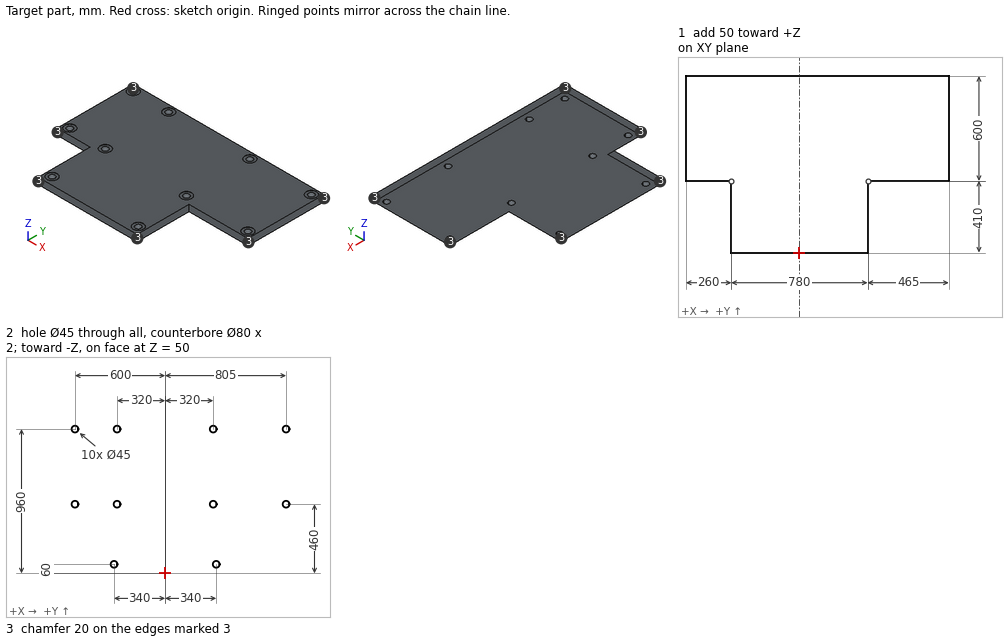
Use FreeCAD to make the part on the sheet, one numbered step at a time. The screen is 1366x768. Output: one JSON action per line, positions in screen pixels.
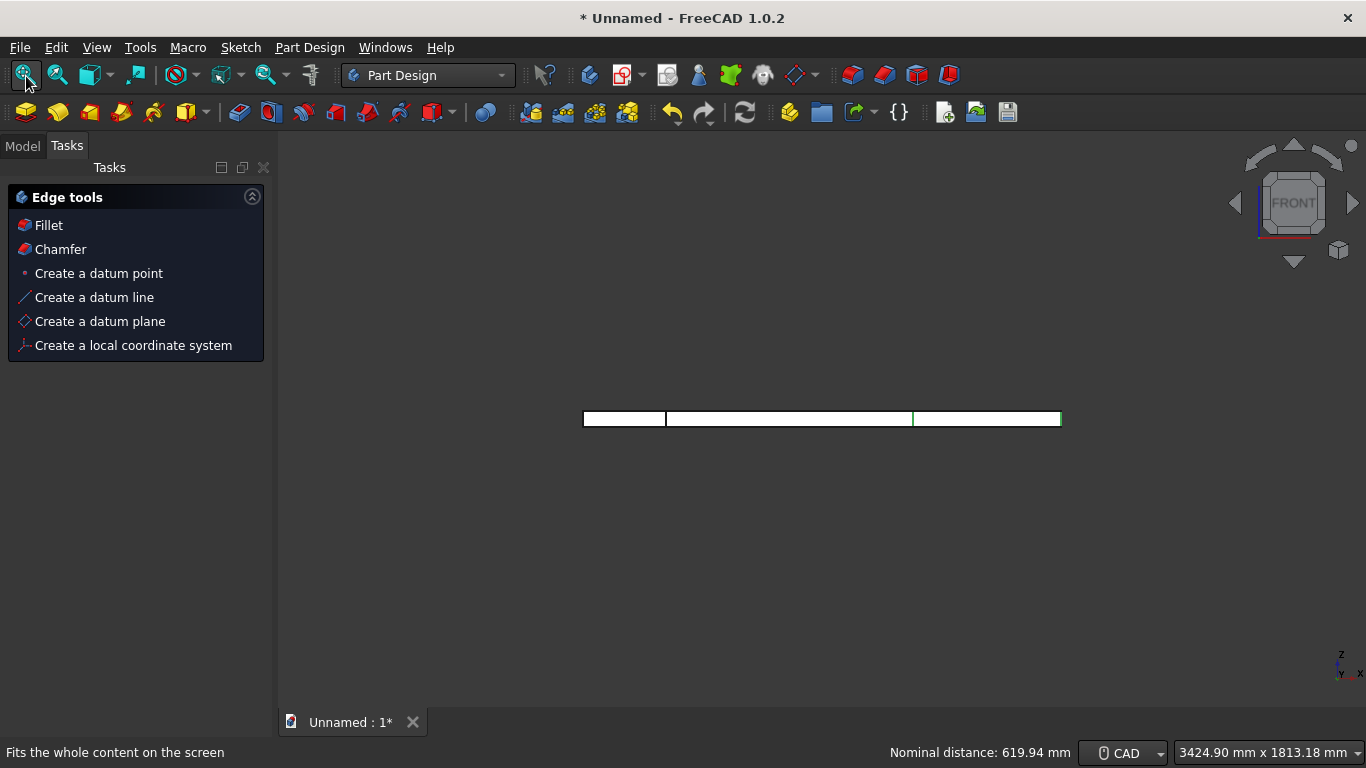
{"action": "key", "text": "v f"}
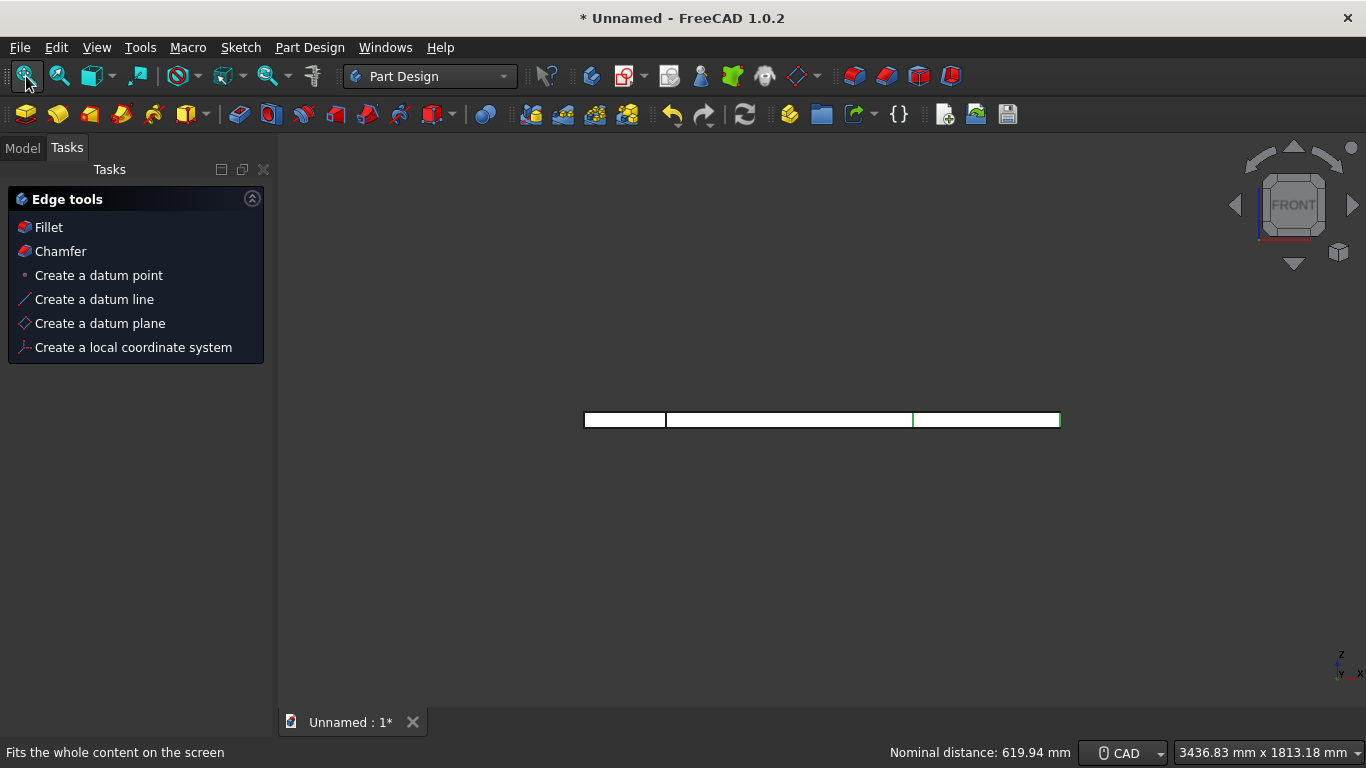
{"action": "left_click", "coordinate": [584, 419], "text": "ctrl"}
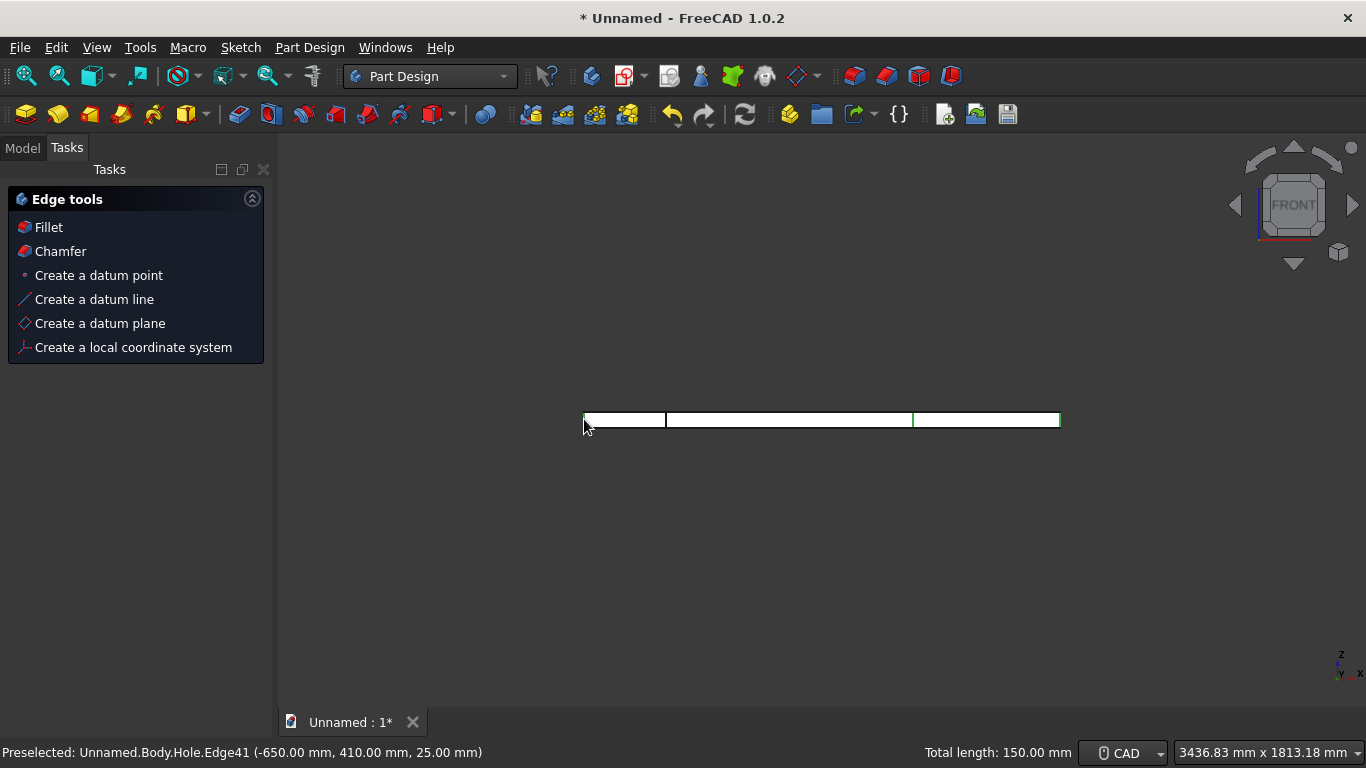
{"action": "scroll", "coordinate": [584, 419], "scroll_direction": "up", "scroll_amount": 5}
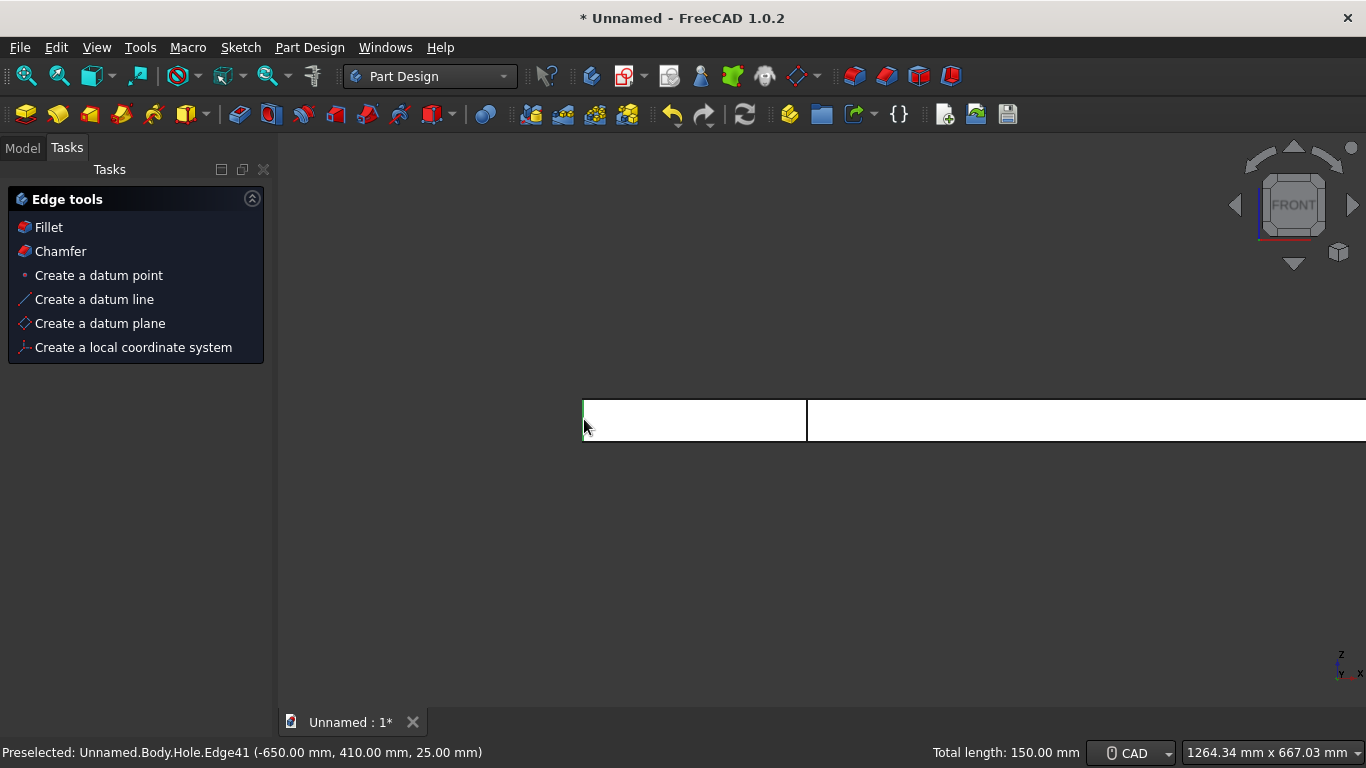
{"action": "left_click", "coordinate": [28, 76]}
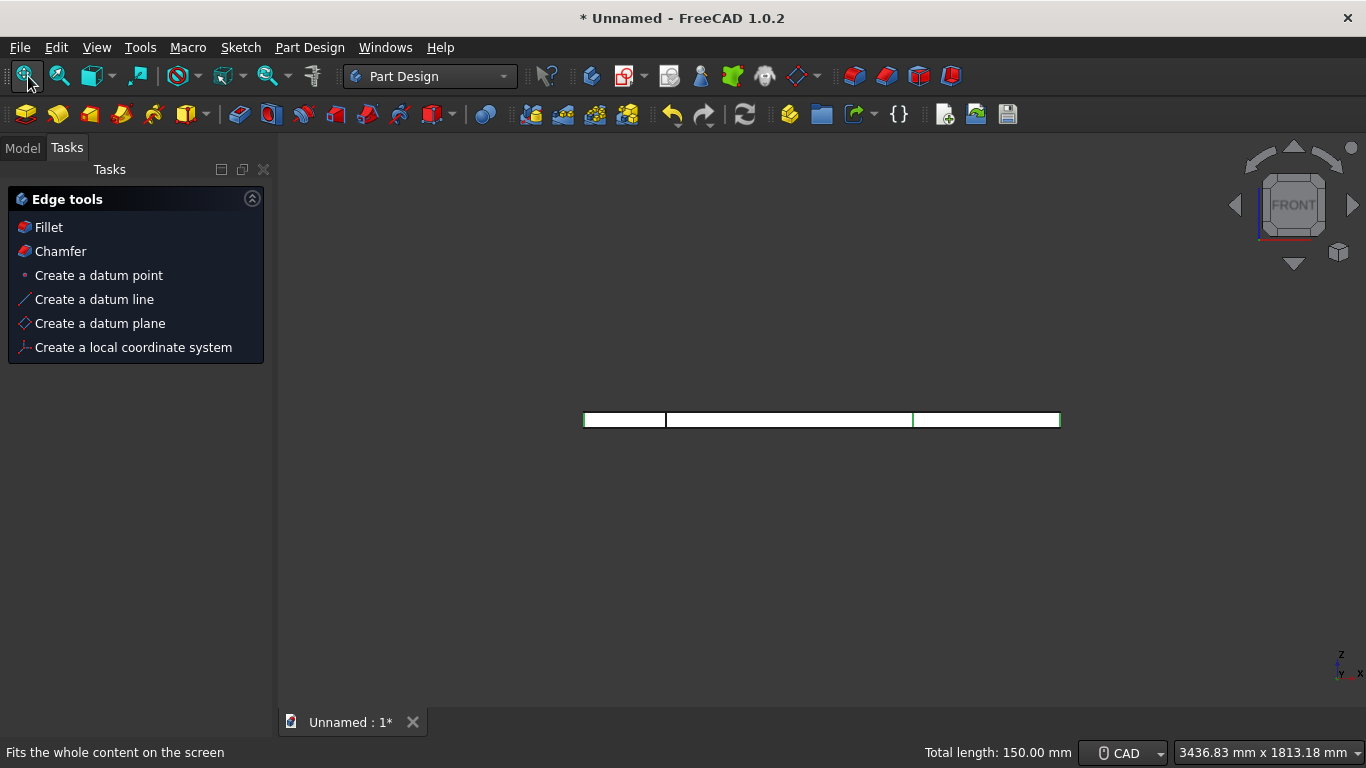
{"action": "key", "text": "3"}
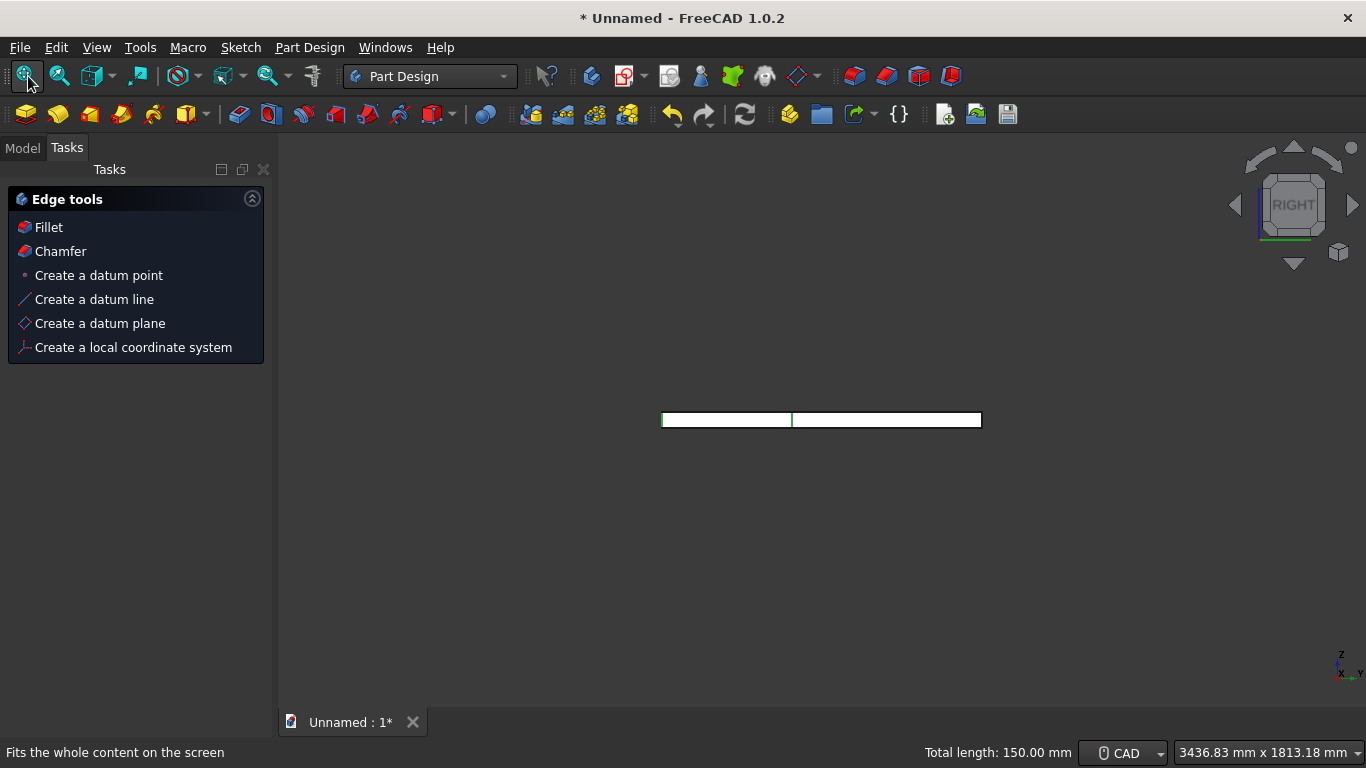
{"action": "key", "text": "v f"}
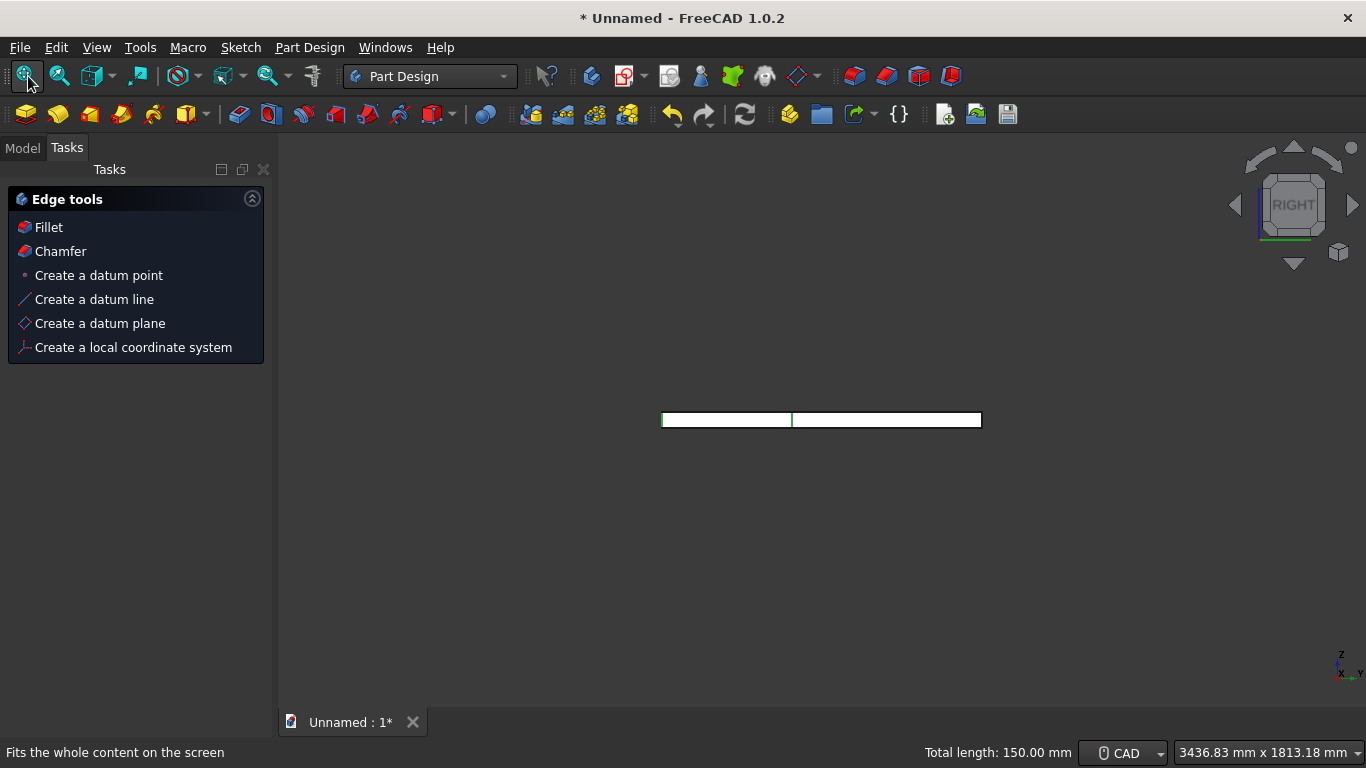
{"action": "left_click", "coordinate": [982, 419], "text": "ctrl"}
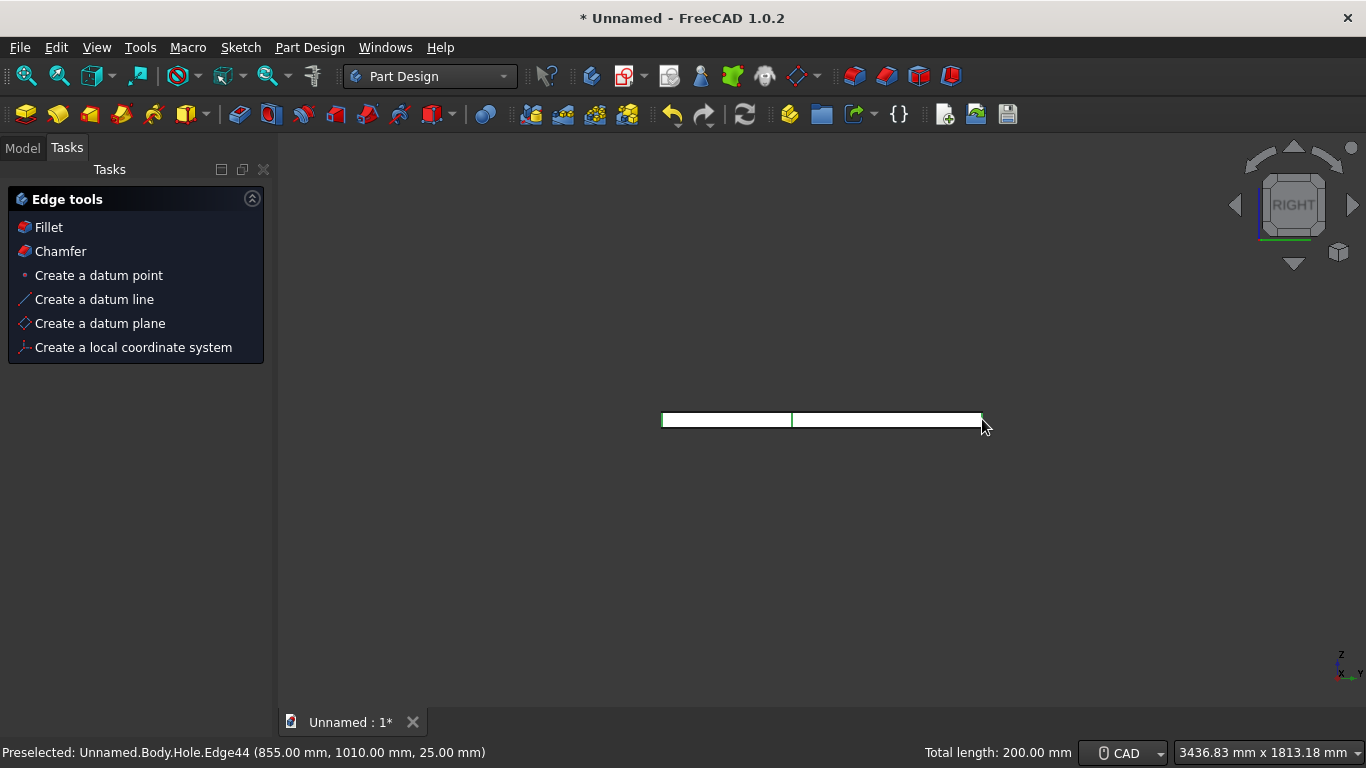
{"action": "scroll", "coordinate": [982, 419], "scroll_direction": "up", "scroll_amount": 5}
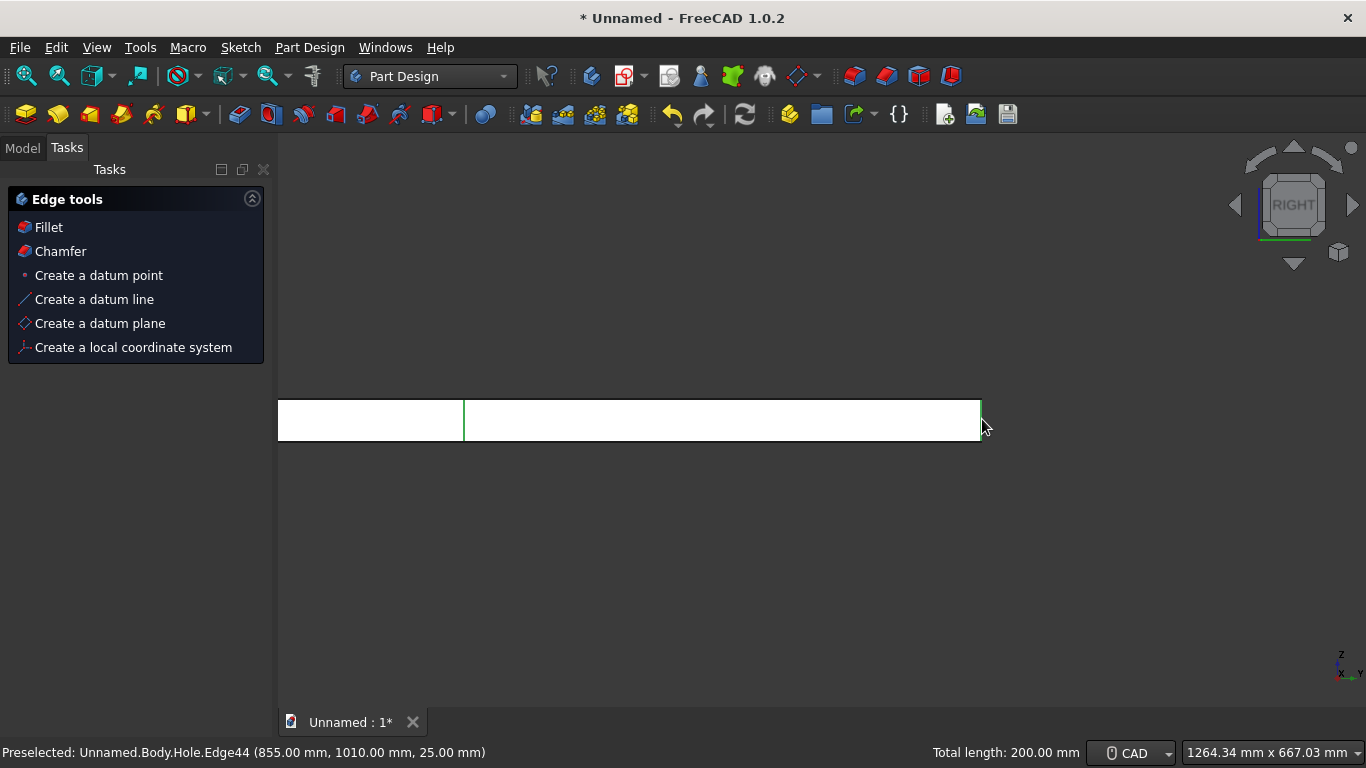
{"action": "left_click", "coordinate": [28, 76]}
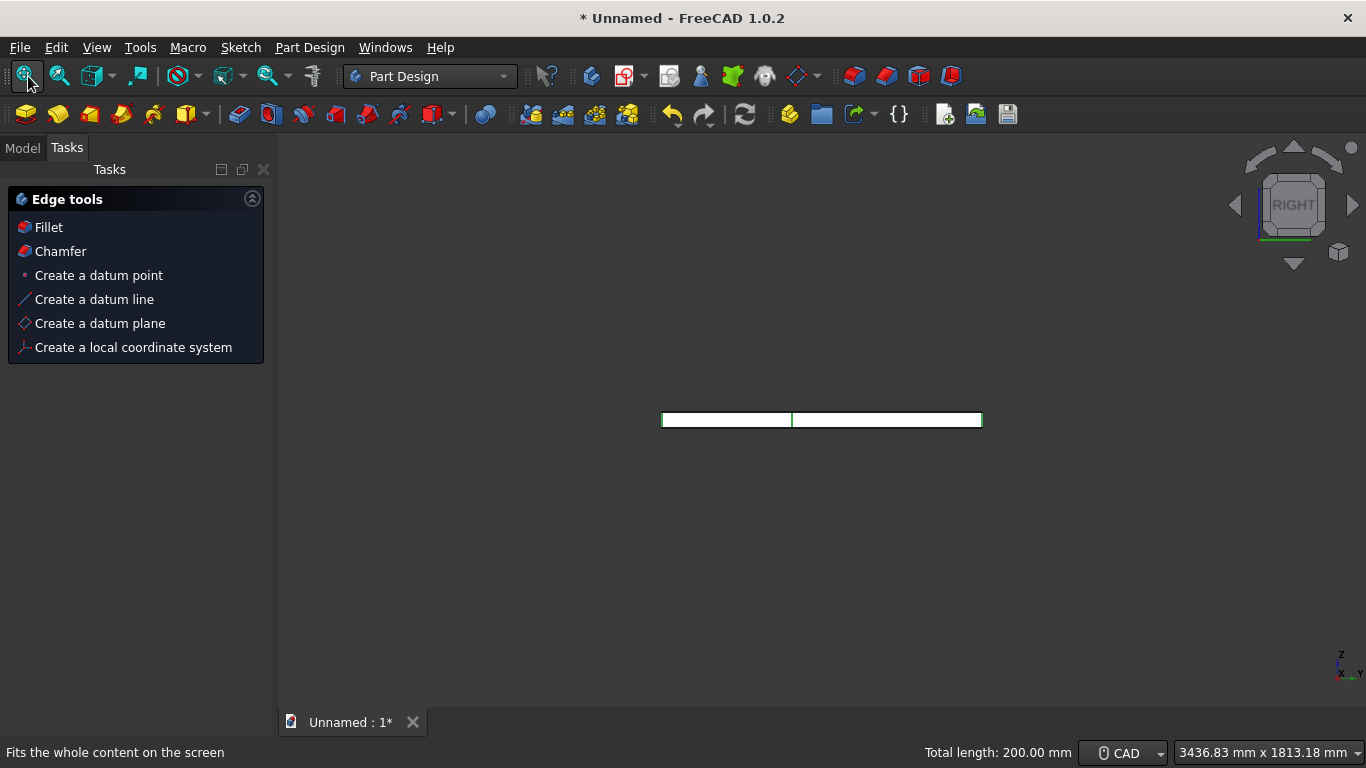
{"action": "key", "text": "5"}